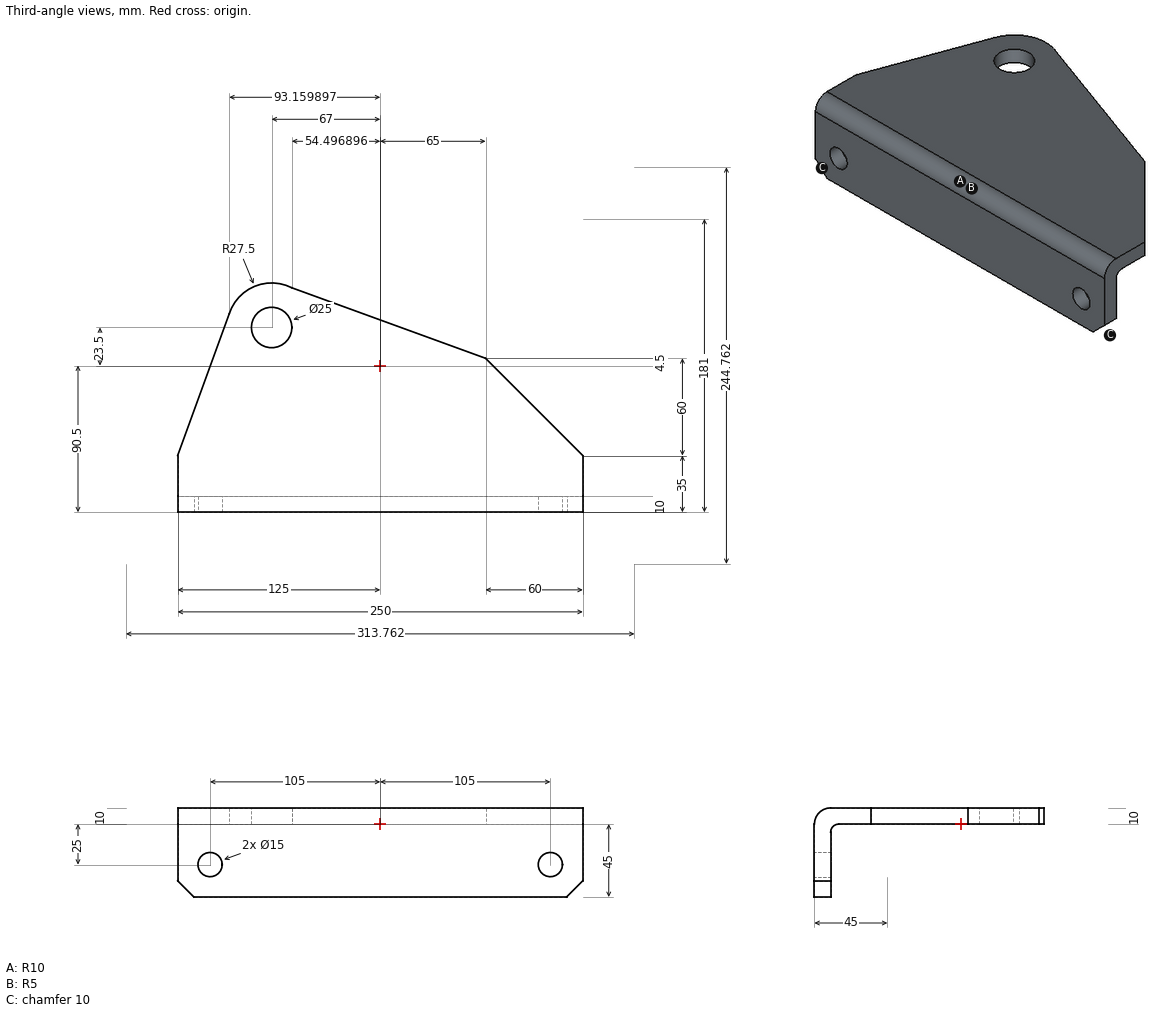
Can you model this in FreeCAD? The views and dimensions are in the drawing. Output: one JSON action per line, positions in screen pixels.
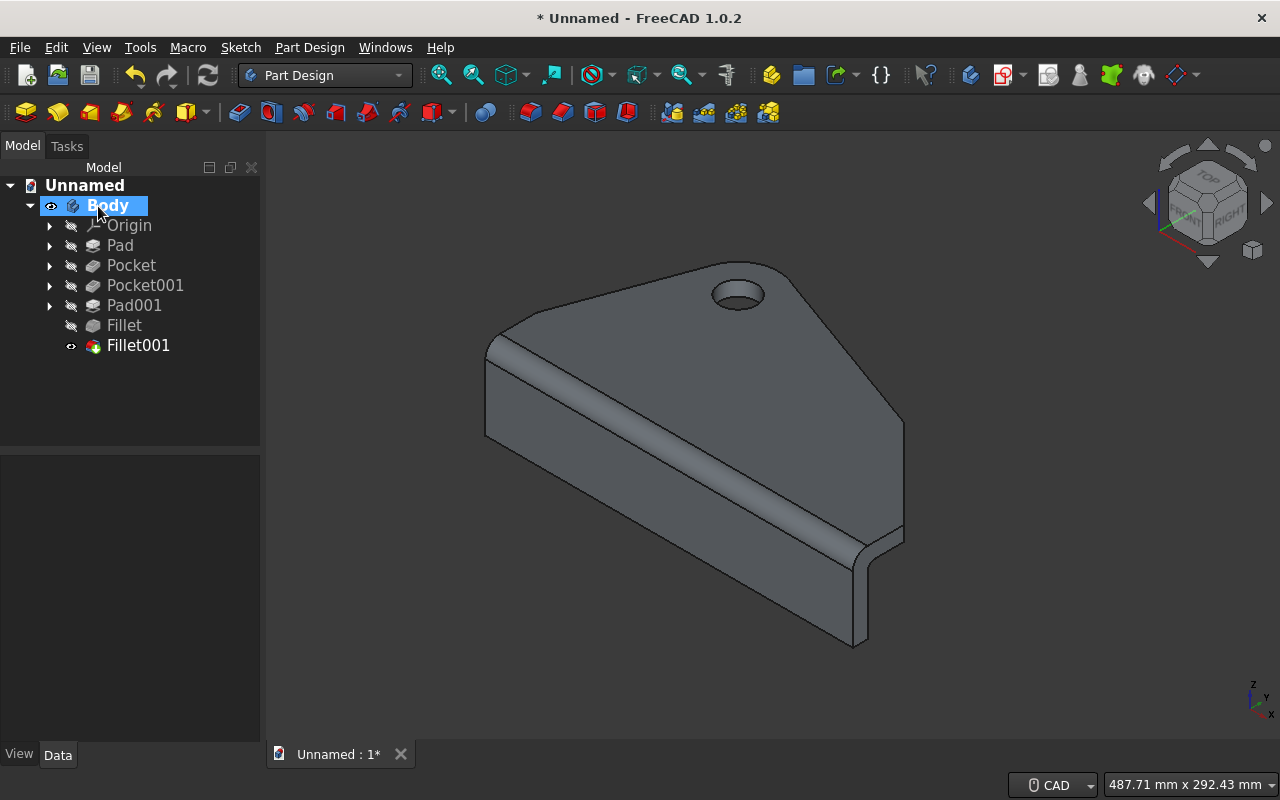
{"action": "left_click", "coordinate": [774, 563]}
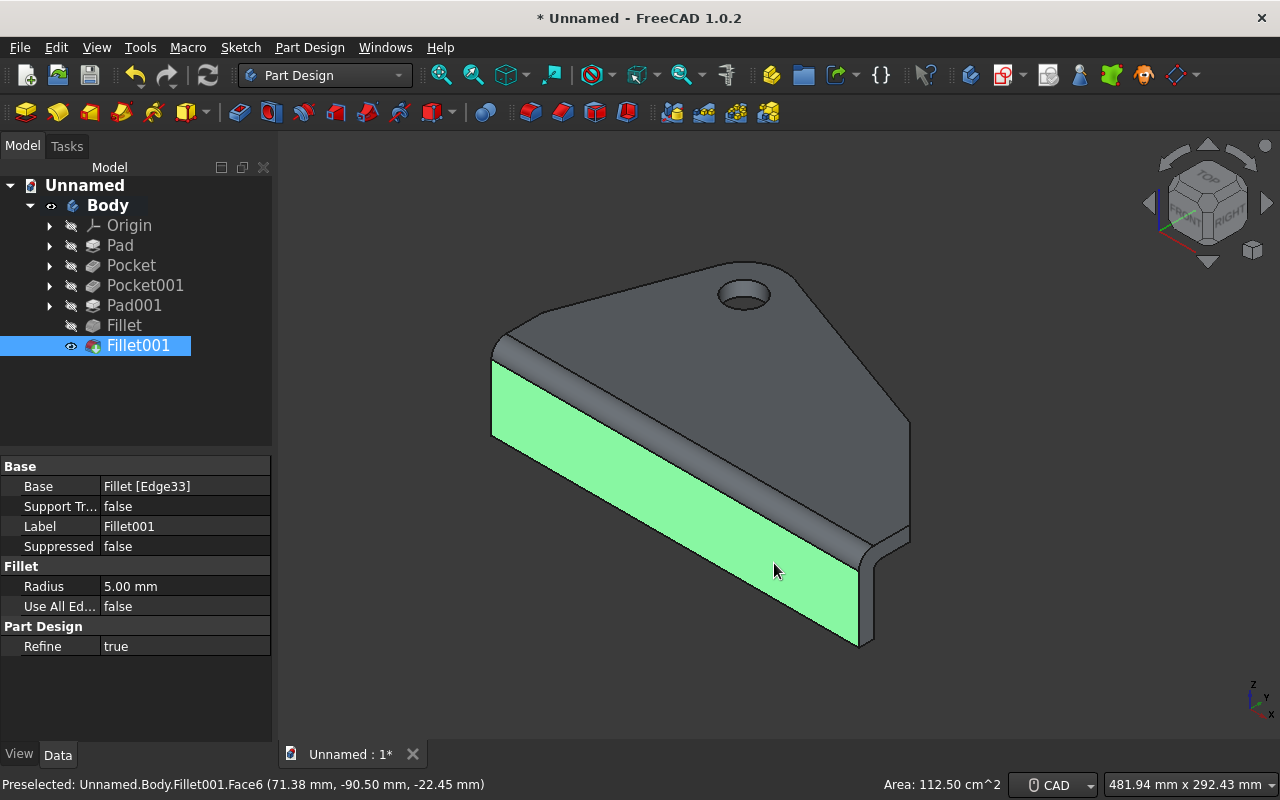
{"action": "left_click", "coordinate": [1004, 76]}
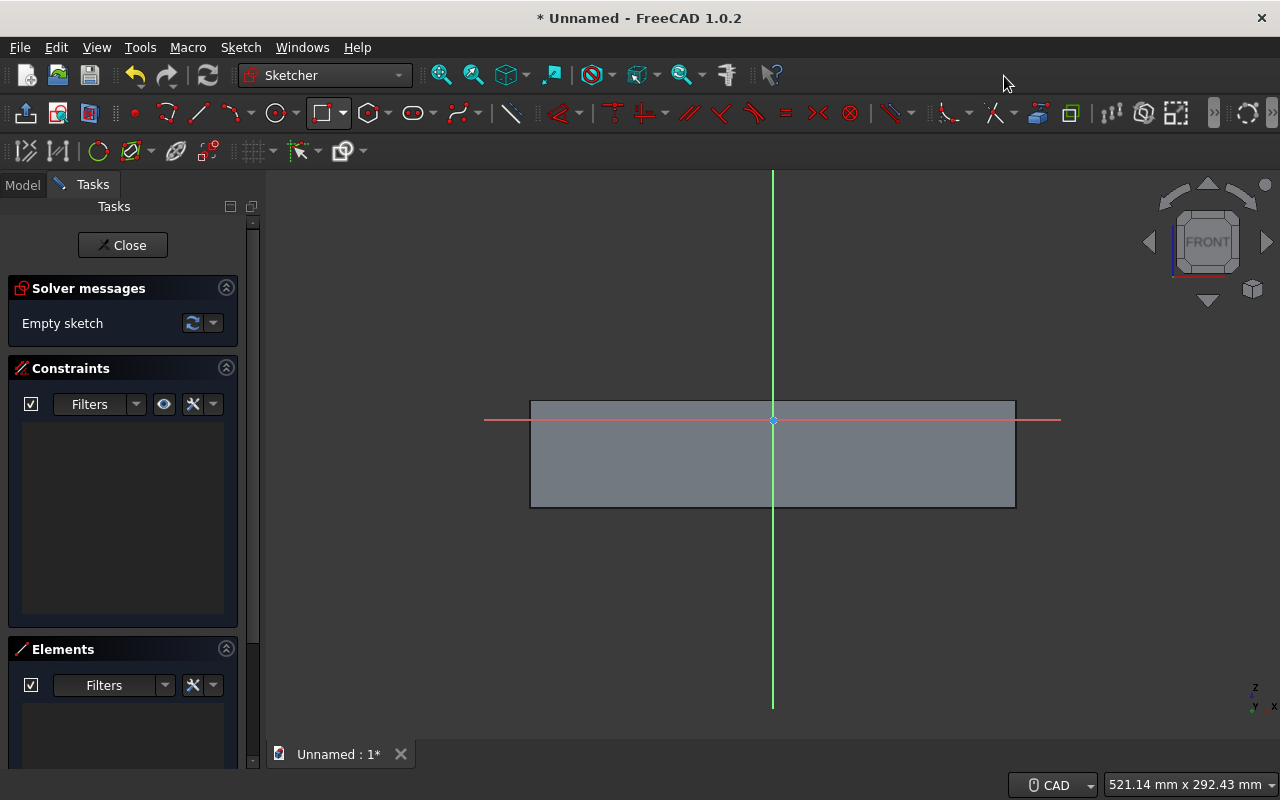
{"action": "left_click", "coordinate": [276, 114]}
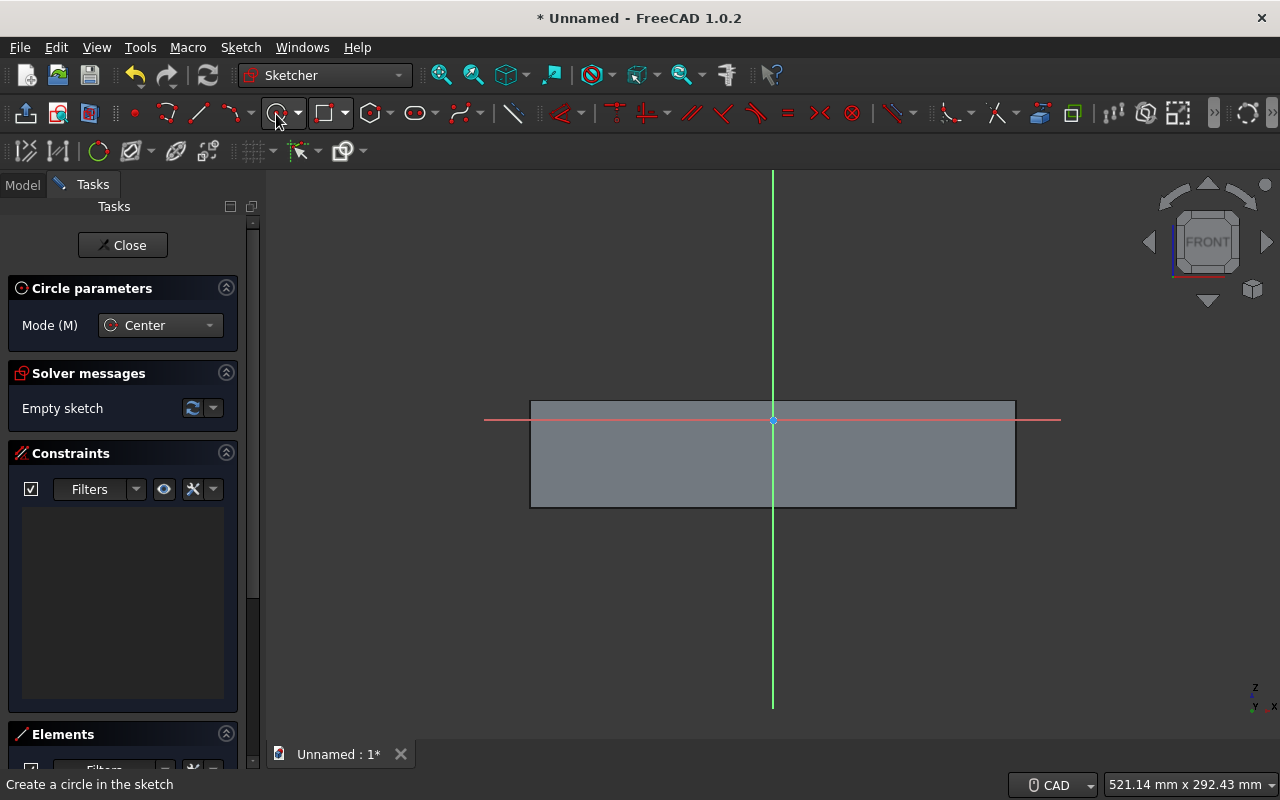
{"action": "scroll", "coordinate": [569, 469], "scroll_direction": "up", "scroll_amount": 3}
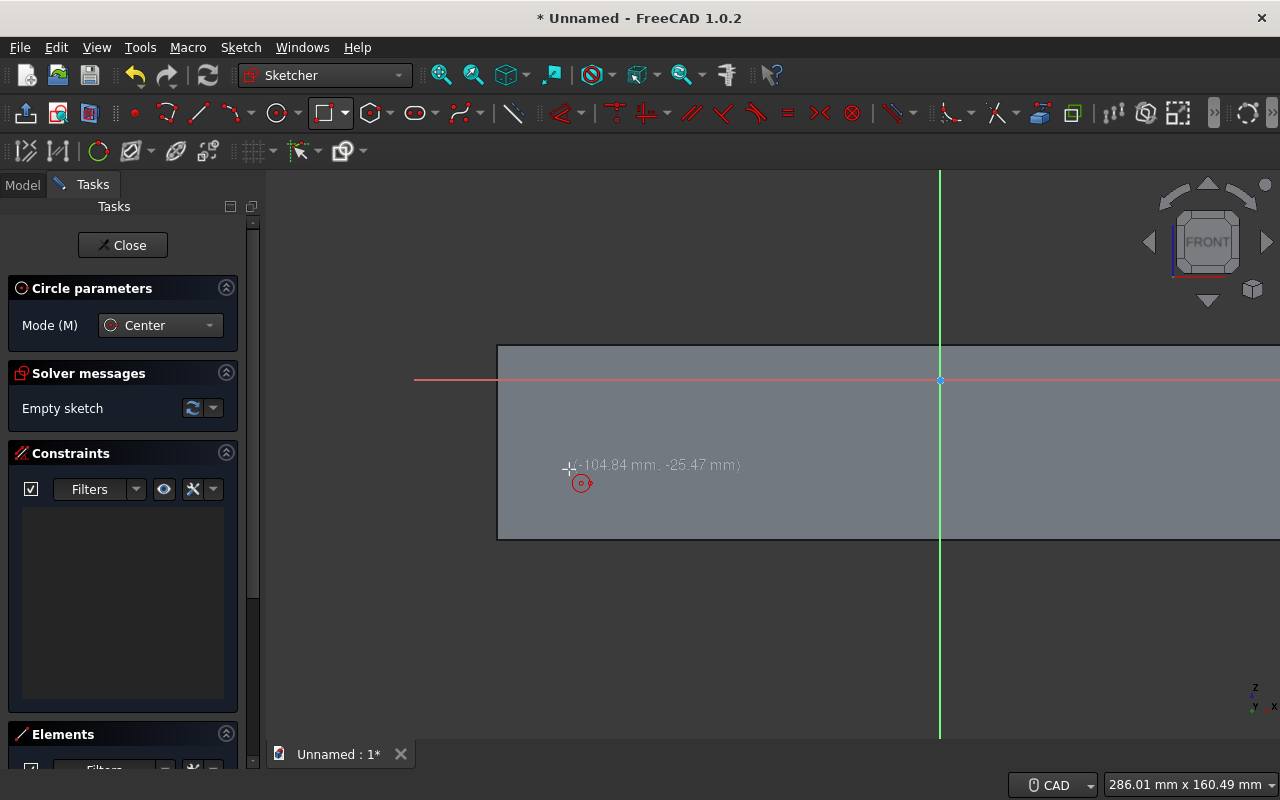
{"action": "left_click", "coordinate": [568, 469]}
{"action": "mouse_move", "coordinate": [587, 450]}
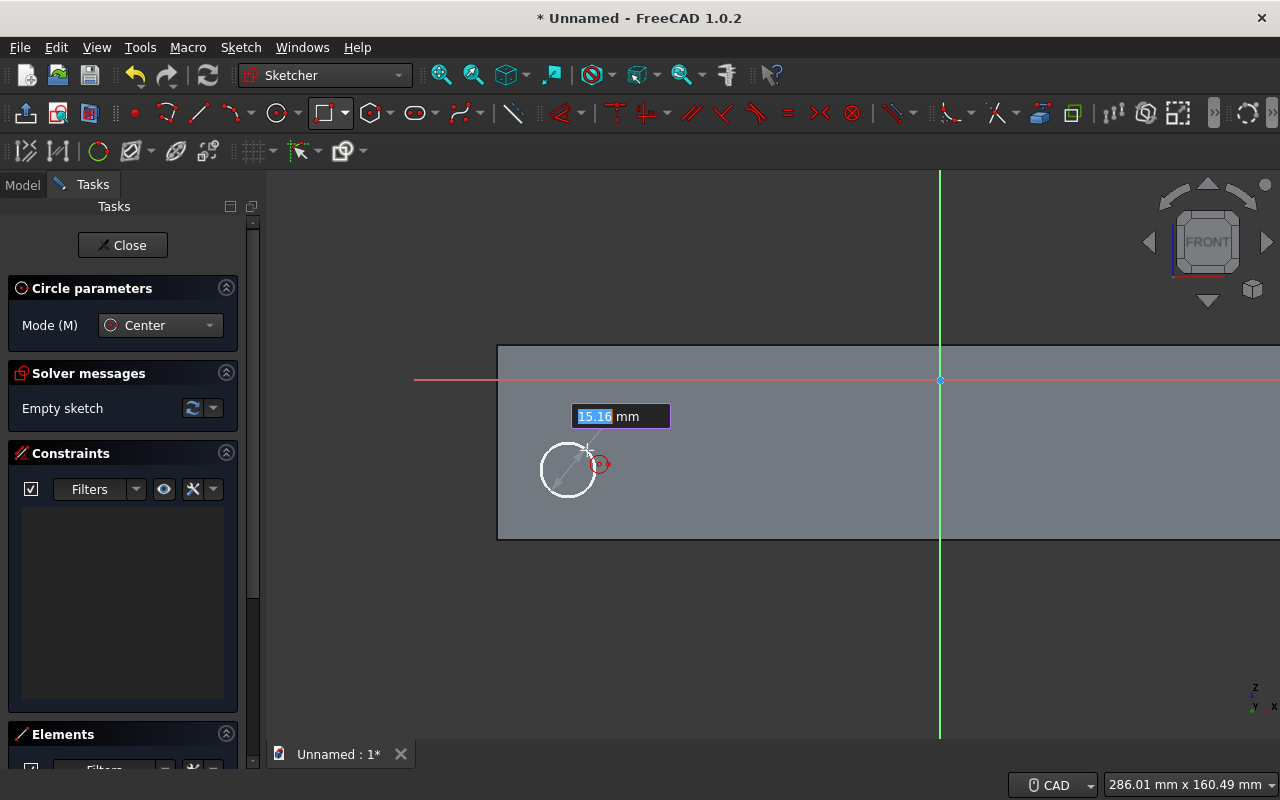
{"action": "type", "text": "15"}
{"action": "key", "text": "Return"}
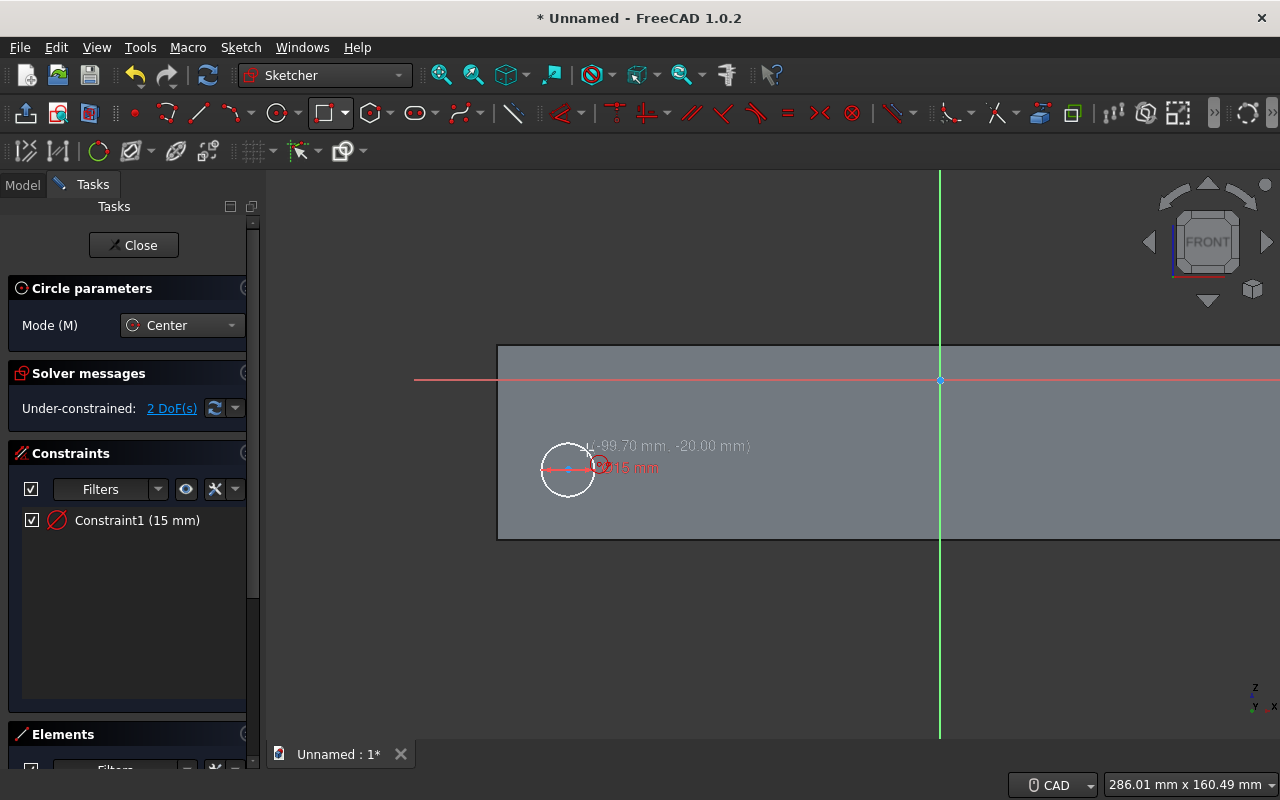
{"action": "scroll", "coordinate": [294, 489], "scroll_direction": "down", "scroll_amount": 2}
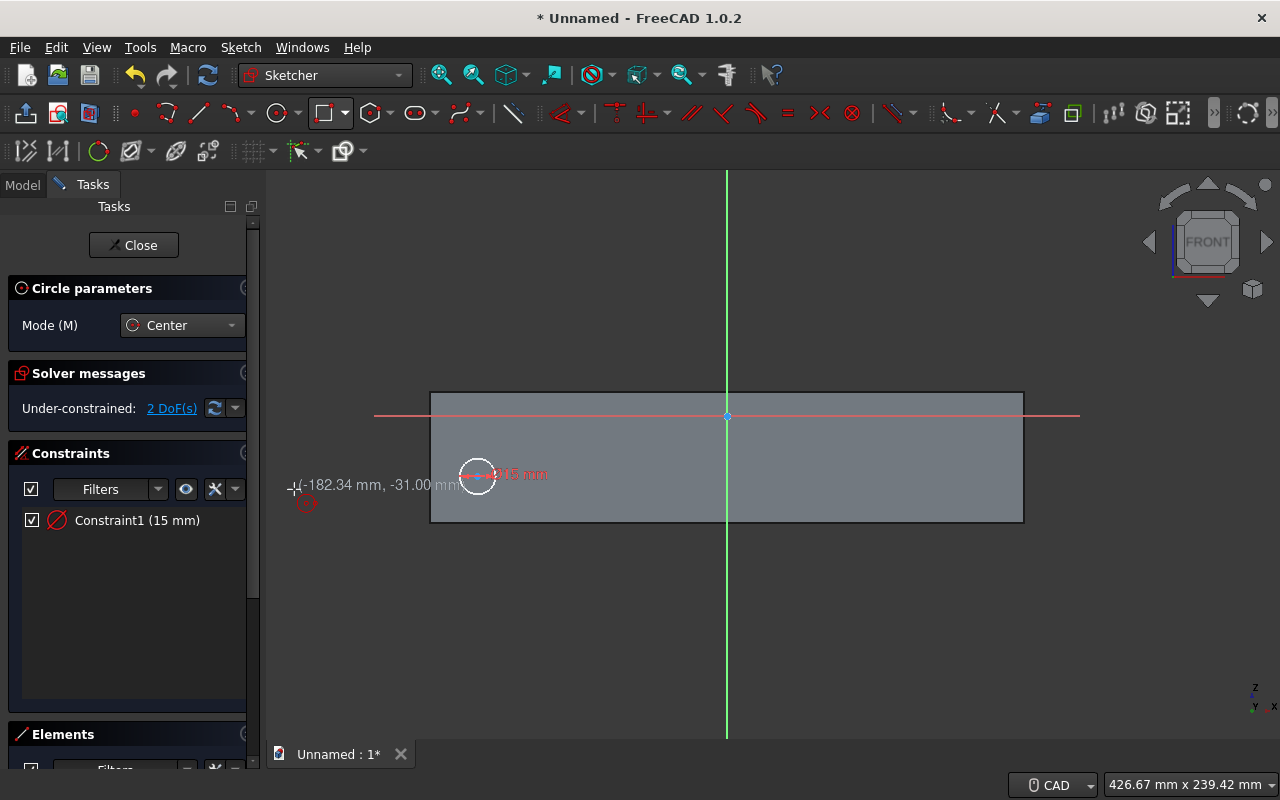
{"action": "scroll", "coordinate": [977, 476], "scroll_direction": "up", "scroll_amount": 2}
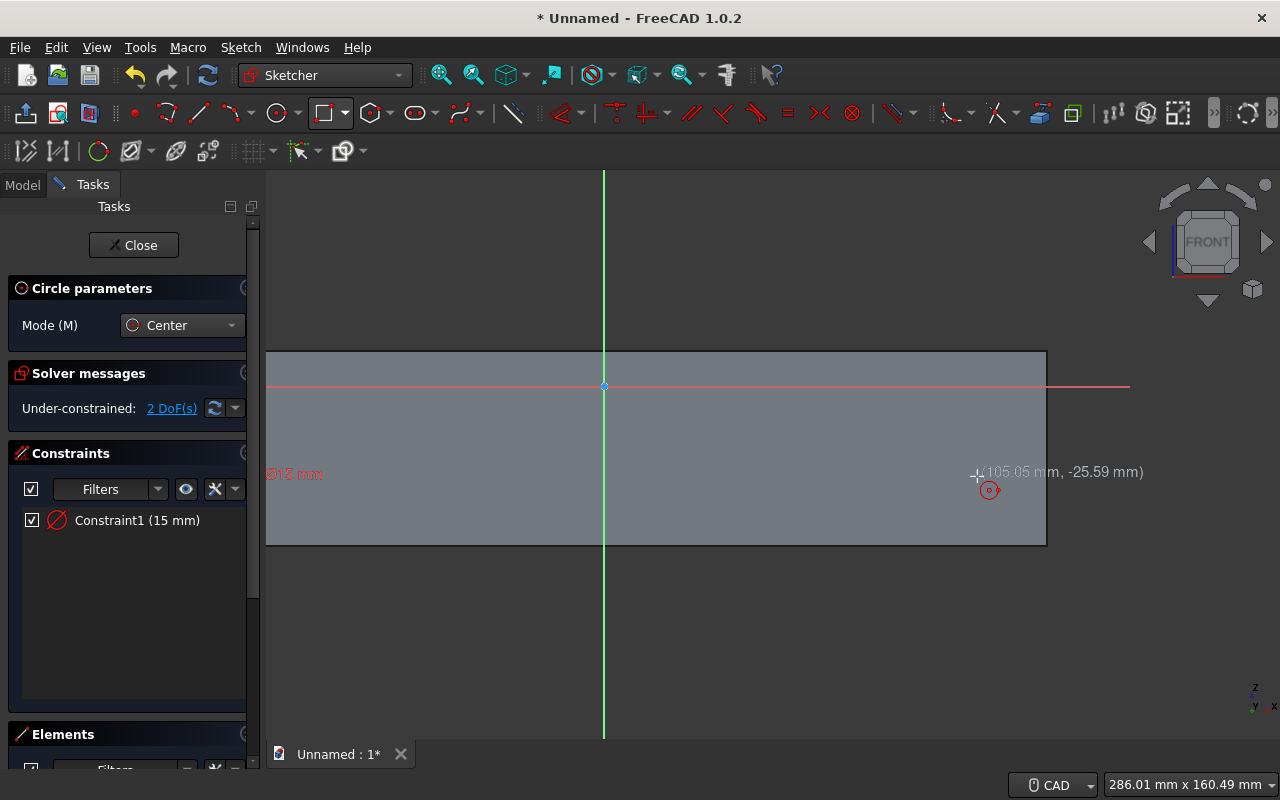
{"action": "left_click", "coordinate": [976, 475]}
{"action": "mouse_move", "coordinate": [995, 456]}